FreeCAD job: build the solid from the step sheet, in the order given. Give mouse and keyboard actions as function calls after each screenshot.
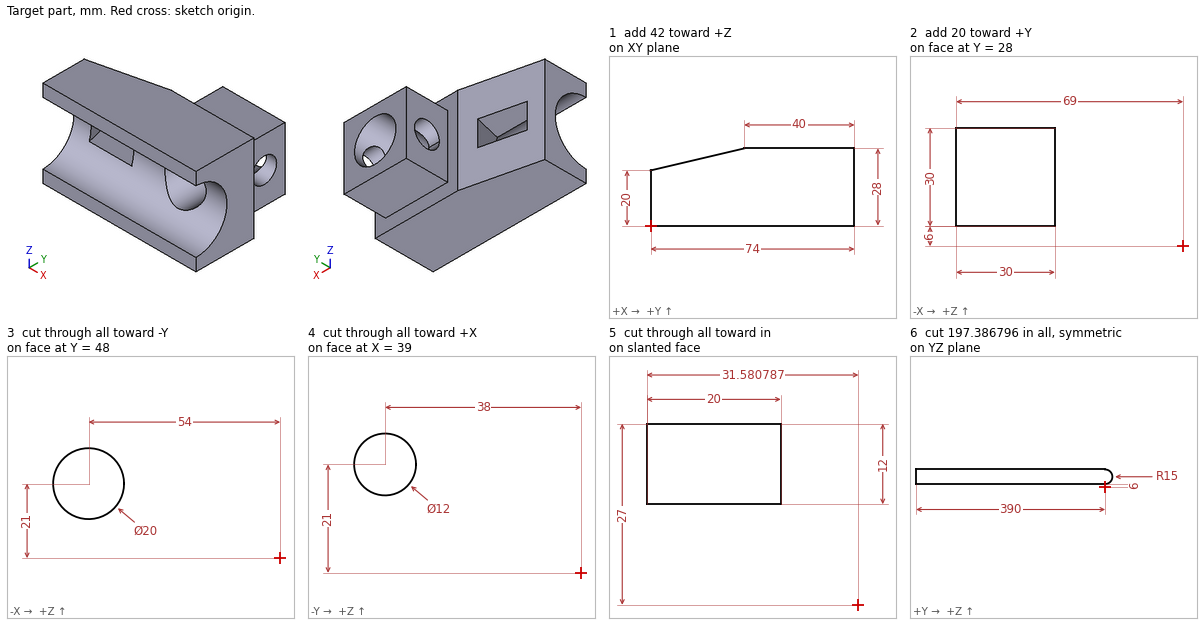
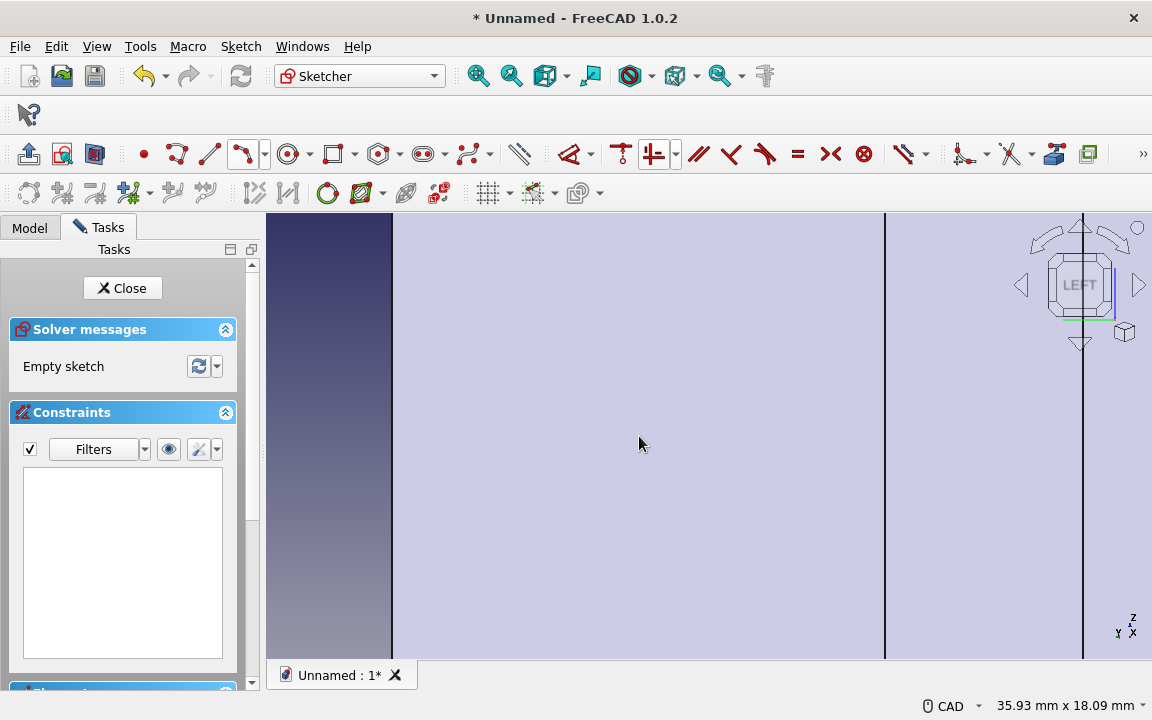
click(288, 154)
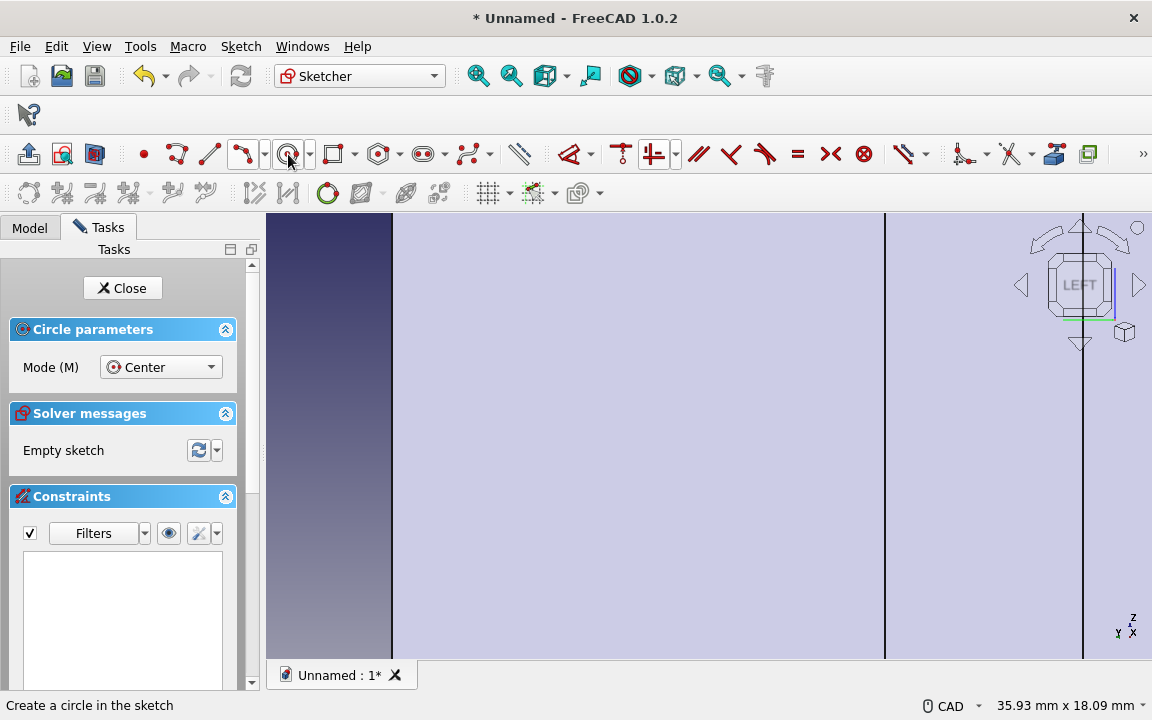
click(639, 434)
move(743, 329)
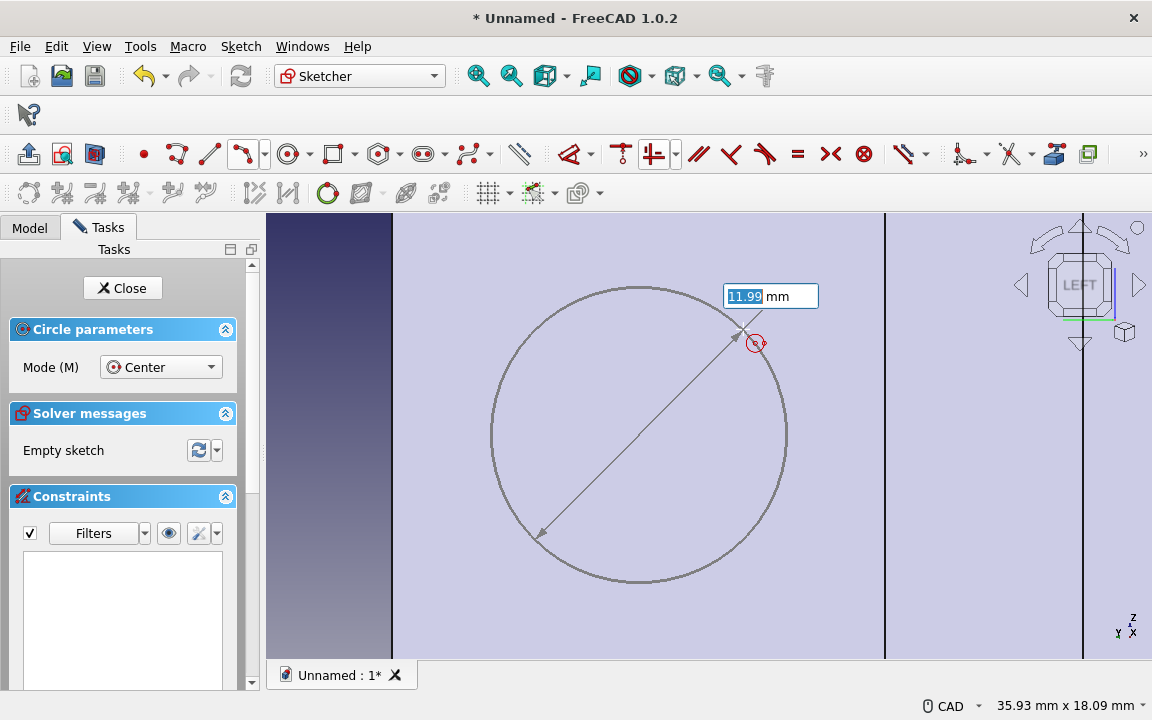
text(12)
key(Return)
key(Escape)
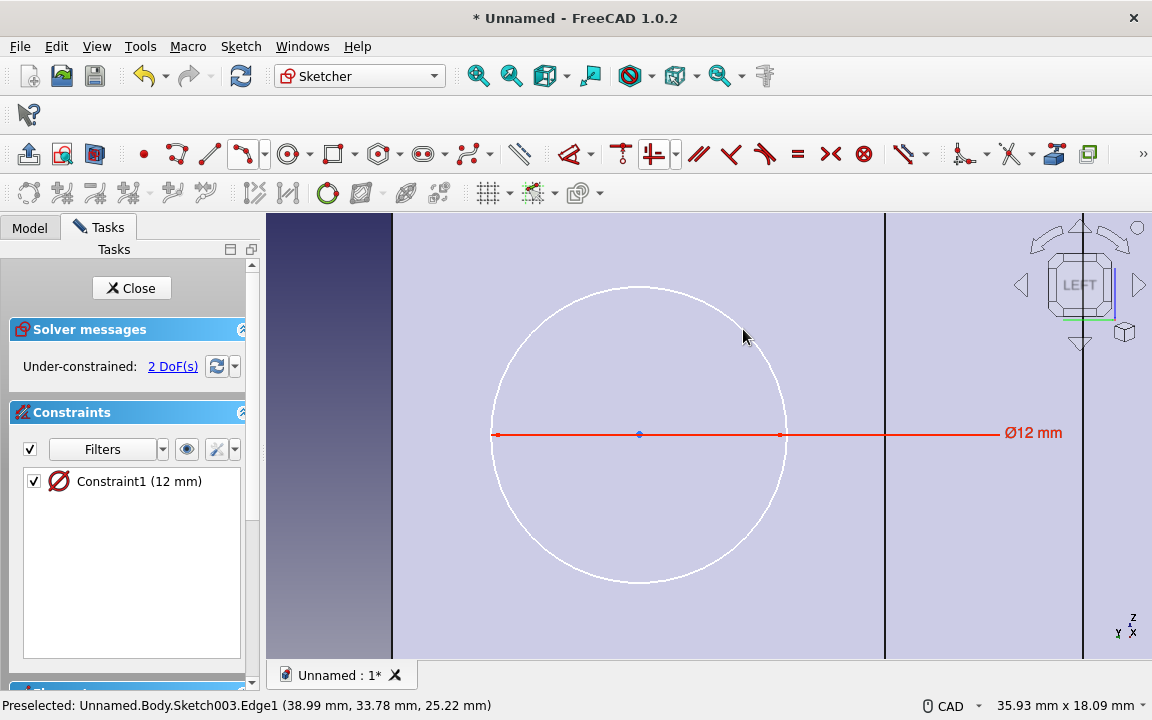
click(568, 154)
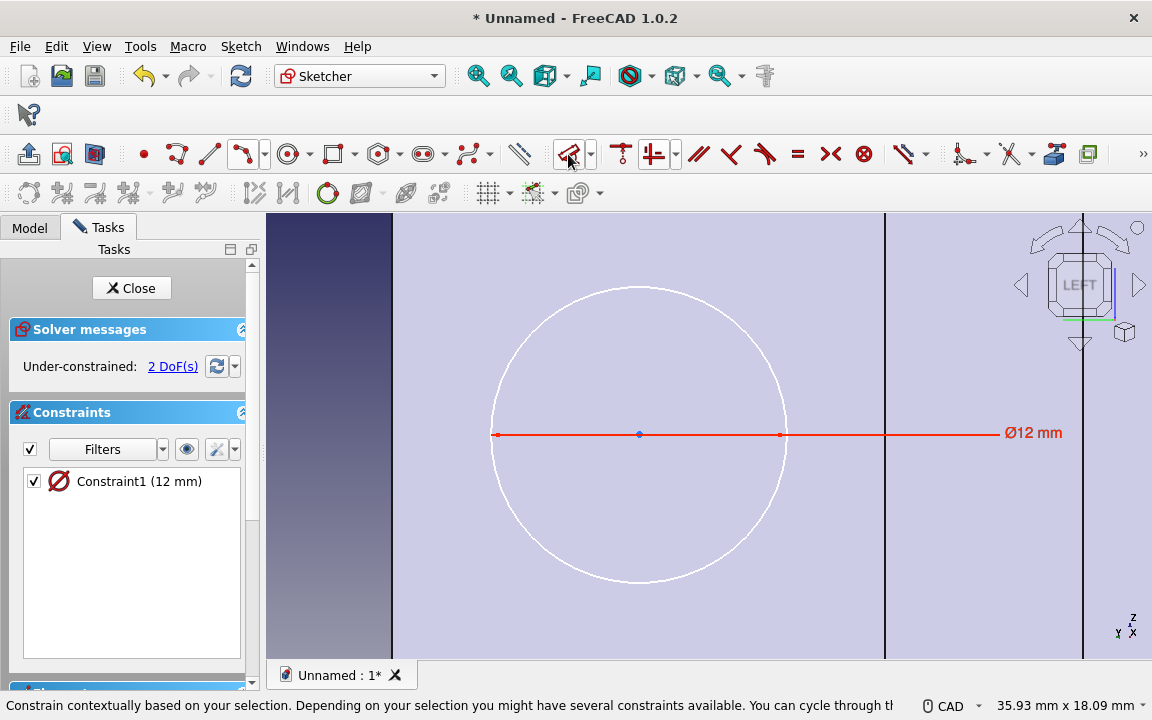
click(639, 435)
click(813, 401)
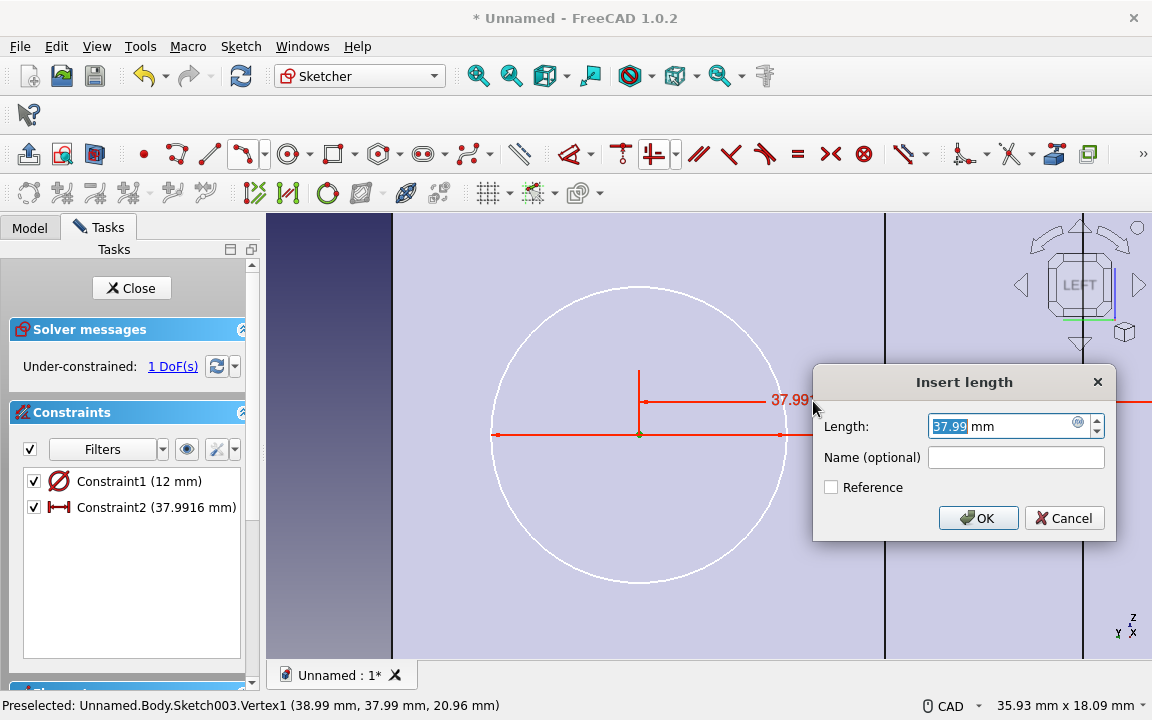
text(38)
key(Return)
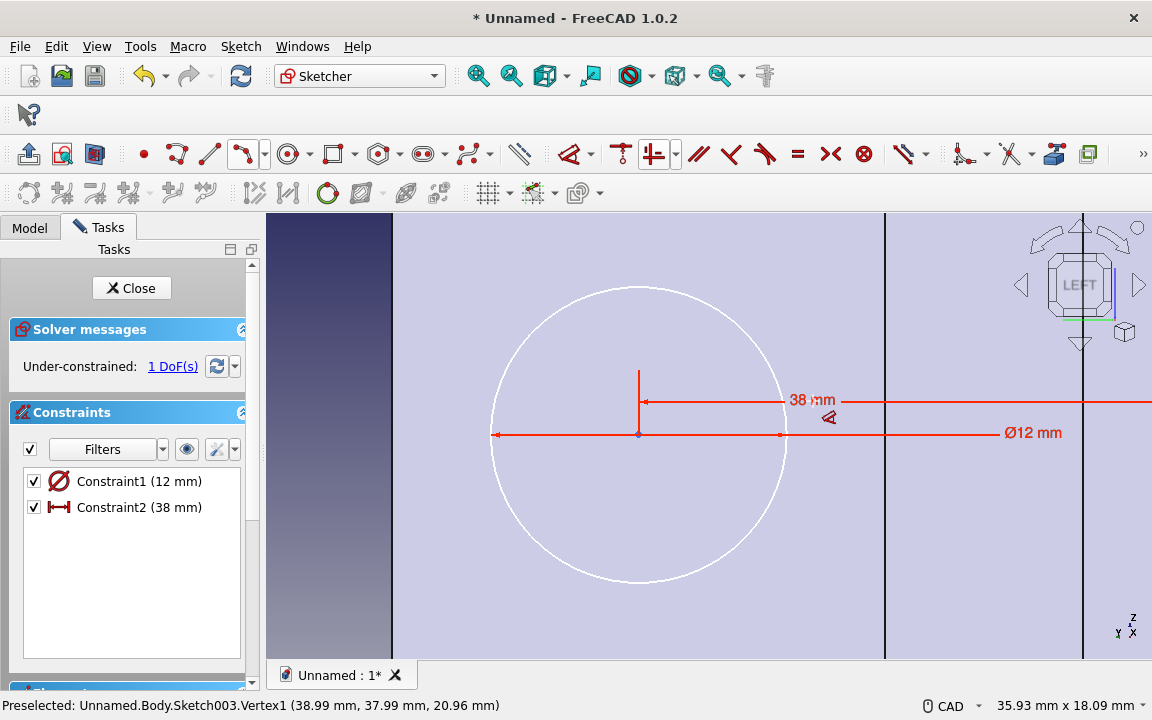
click(639, 435)
click(605, 533)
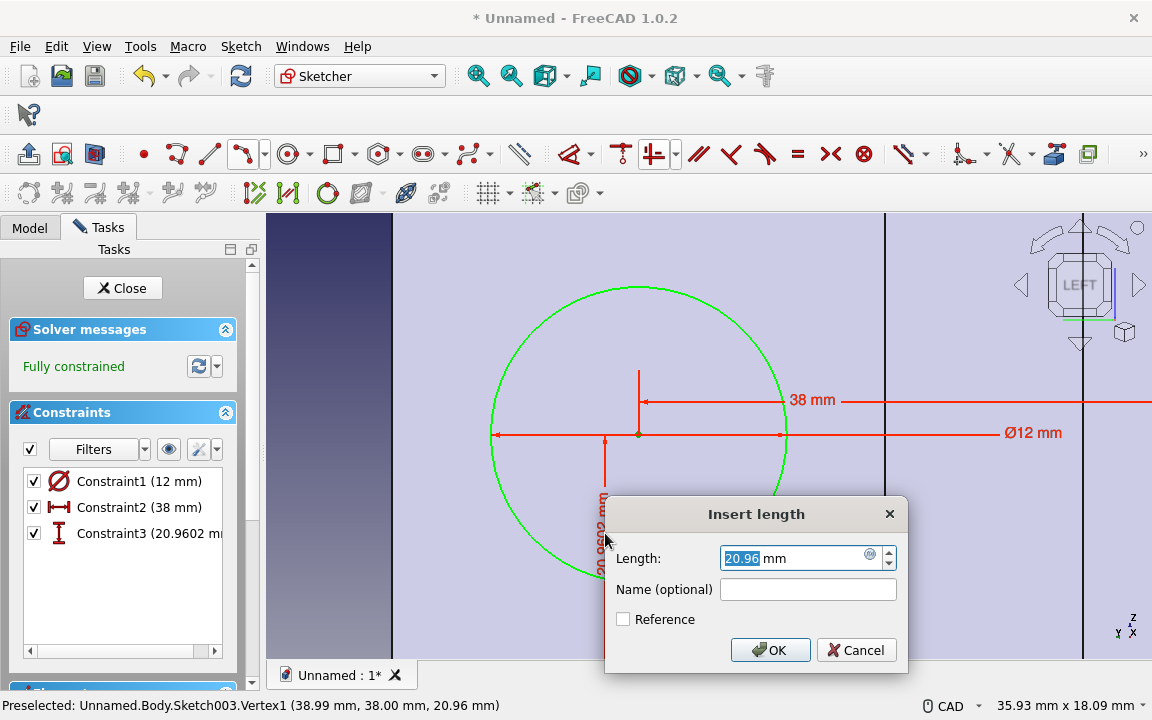
text(21)
key(Return)
key(Escape)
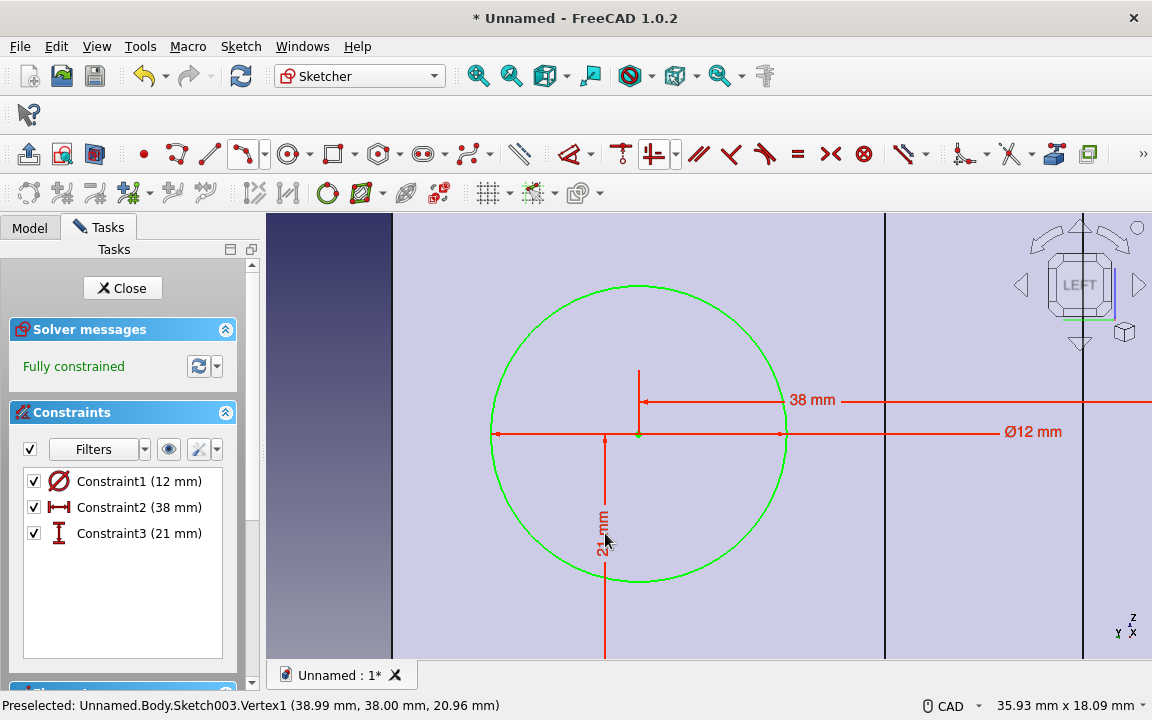
click(123, 288)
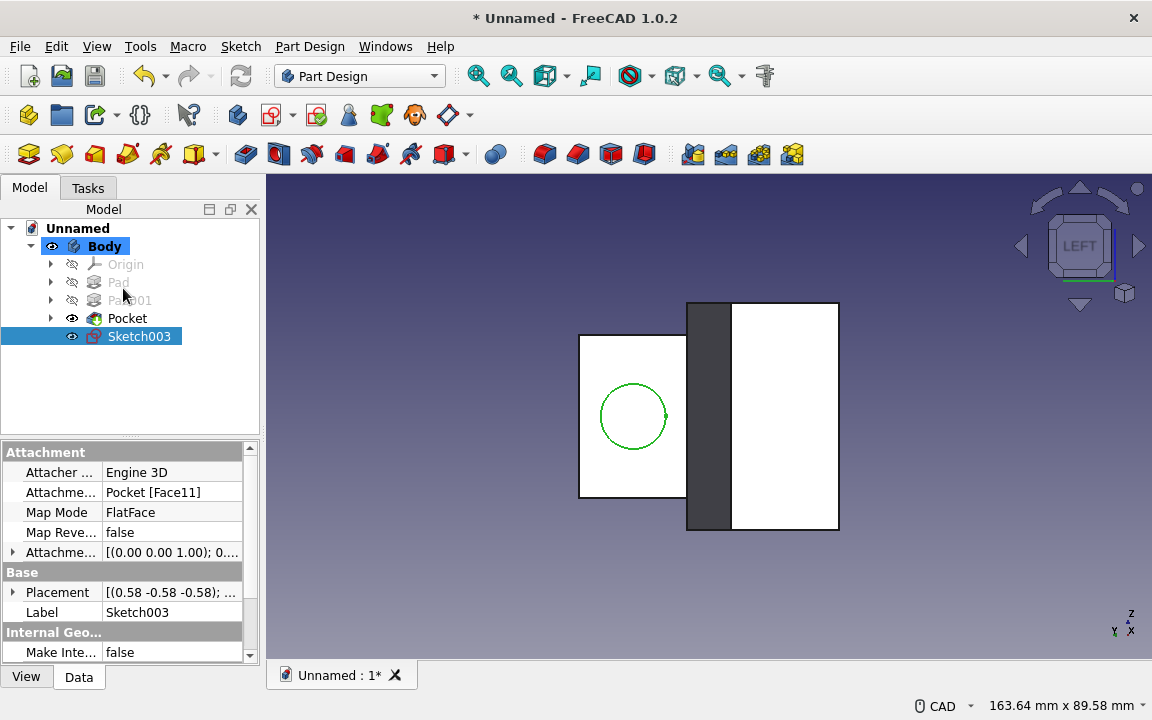
click(246, 154)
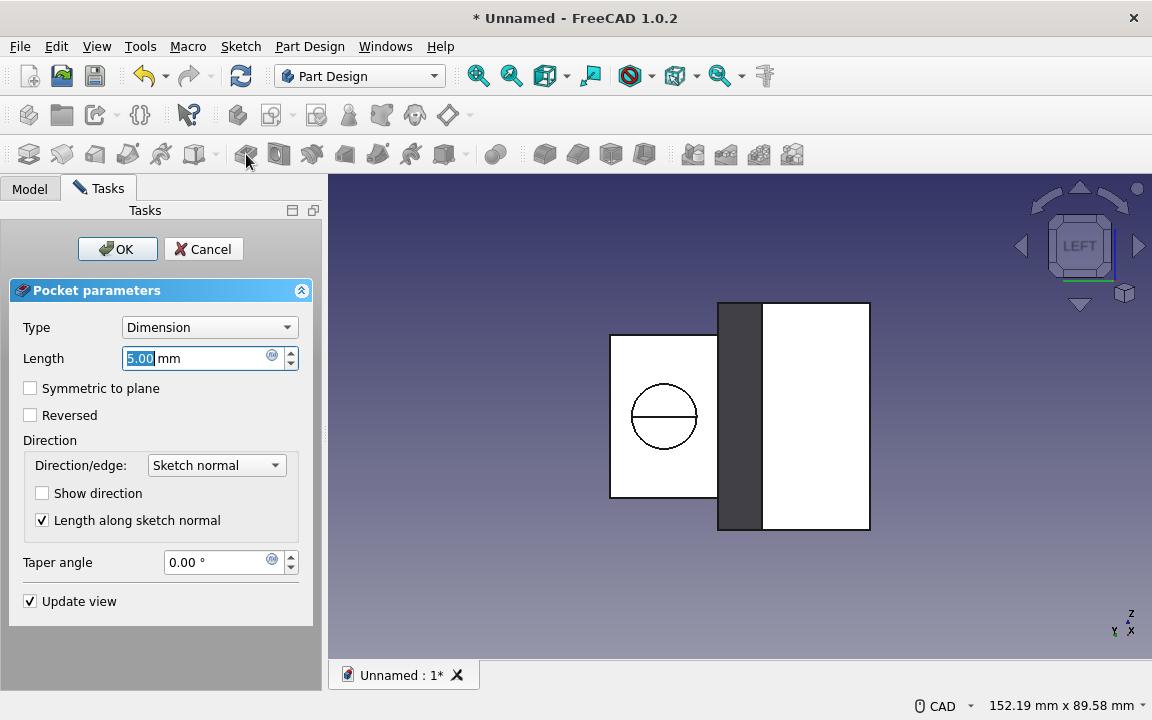
click(210, 328)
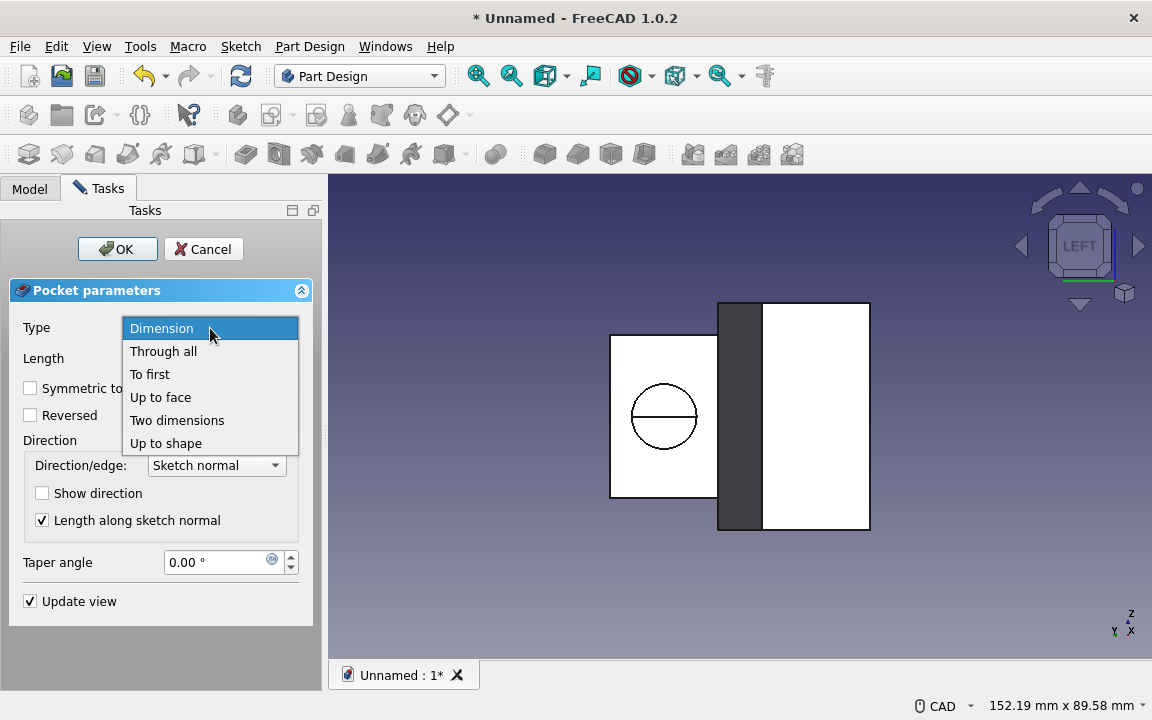
click(208, 352)